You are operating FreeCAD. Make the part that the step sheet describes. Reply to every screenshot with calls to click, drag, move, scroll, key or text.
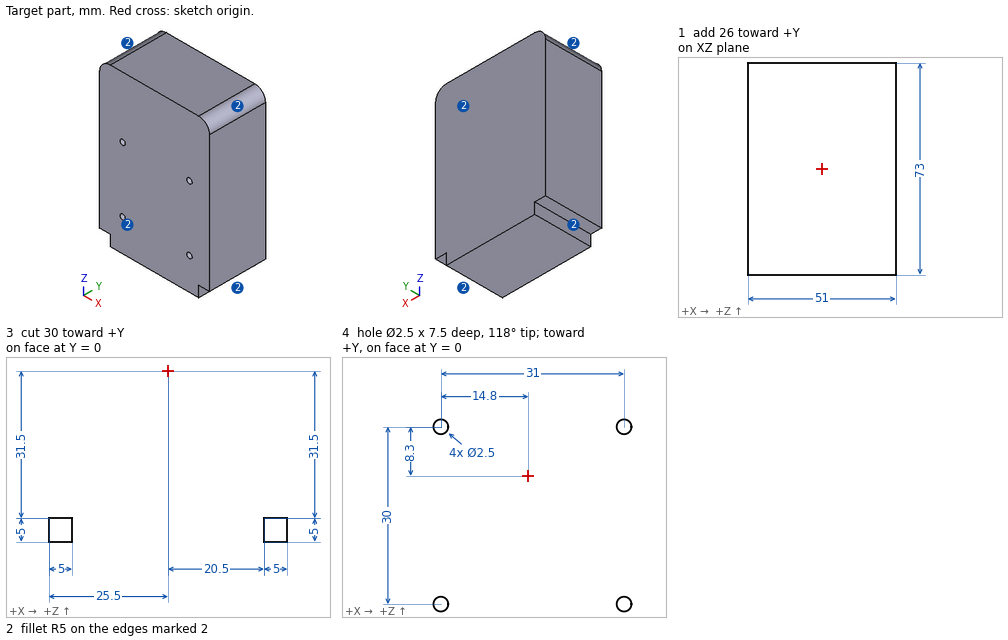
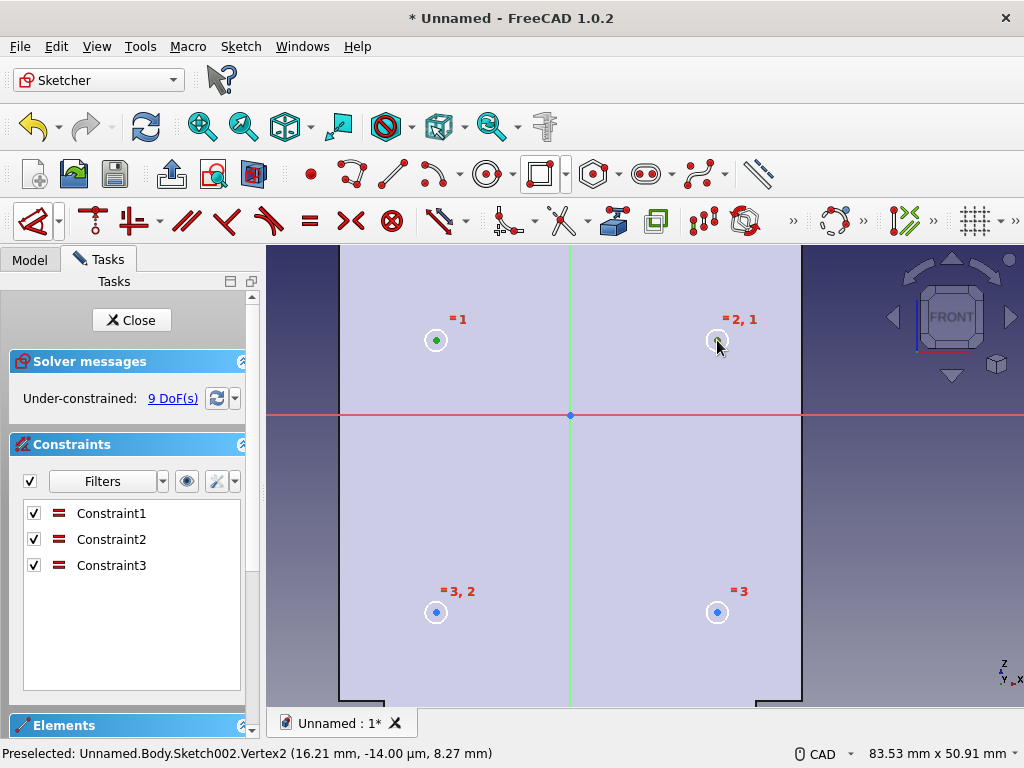
click(160, 222)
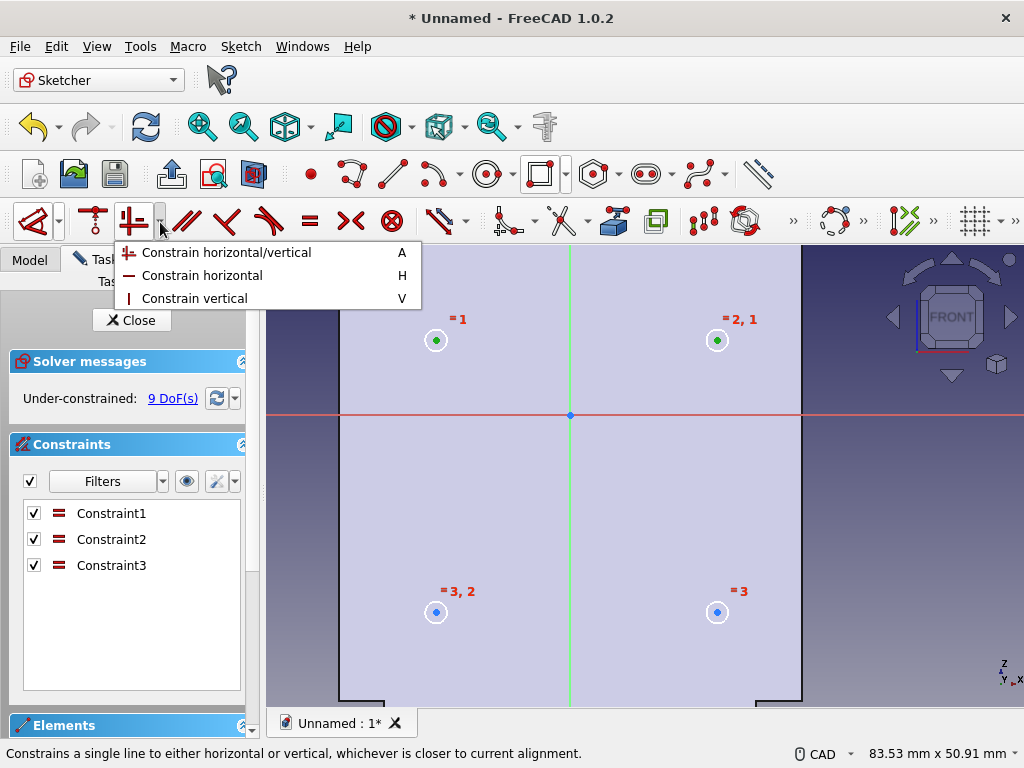
click(268, 276)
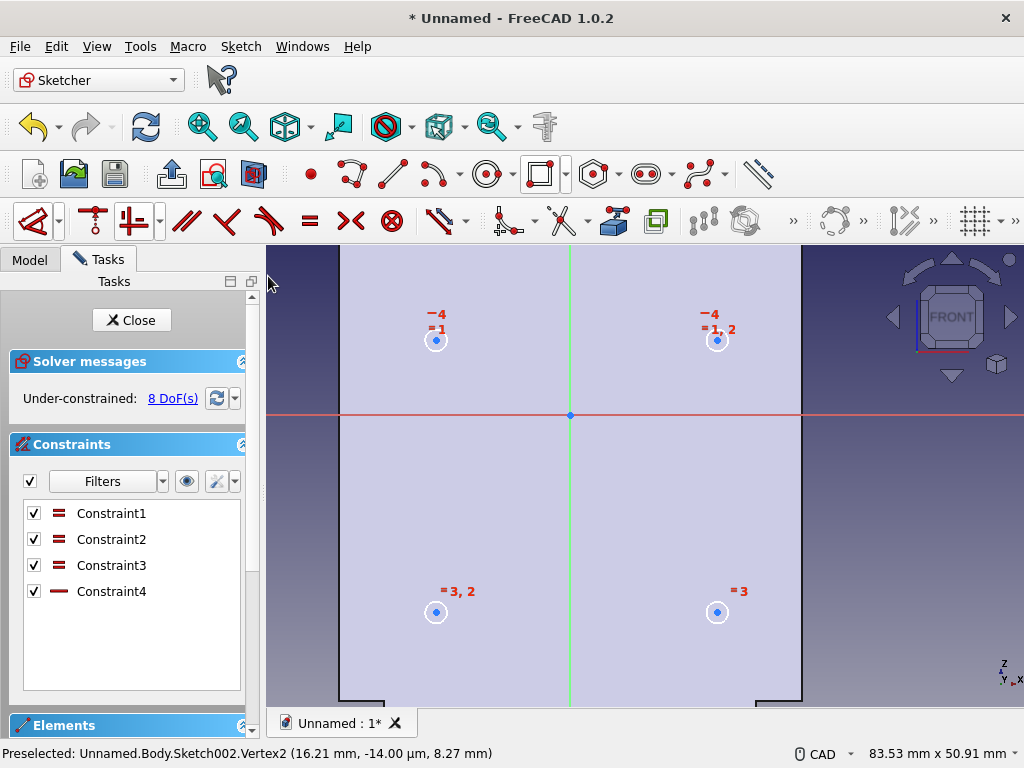
click(436, 340)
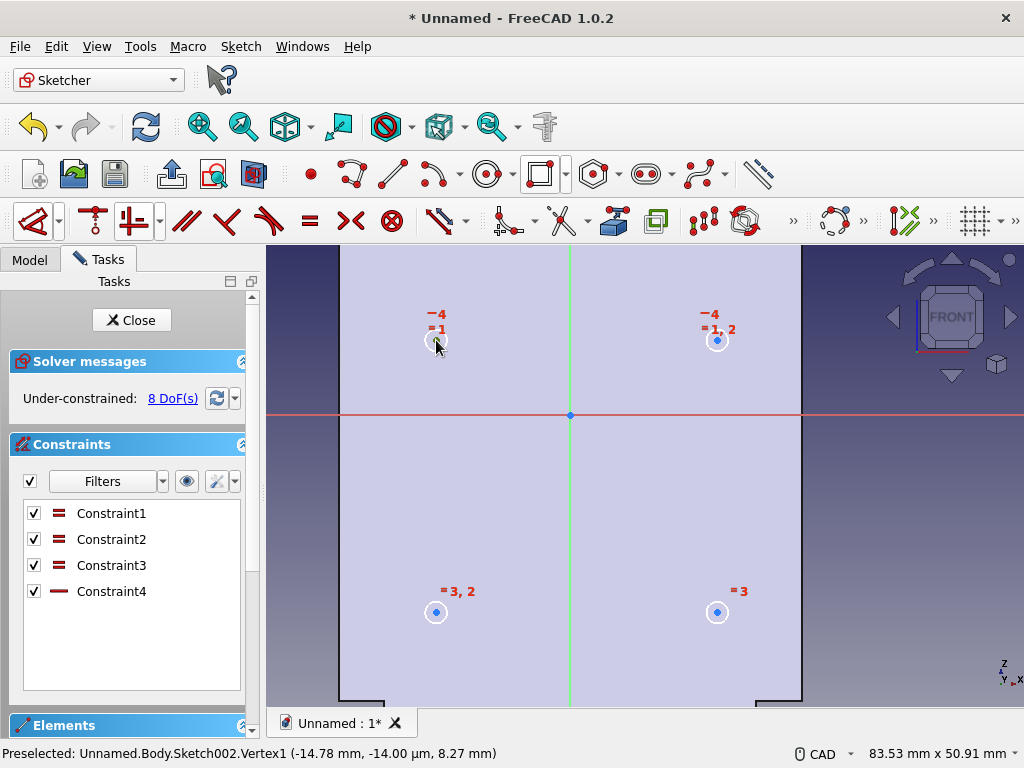
click(436, 613)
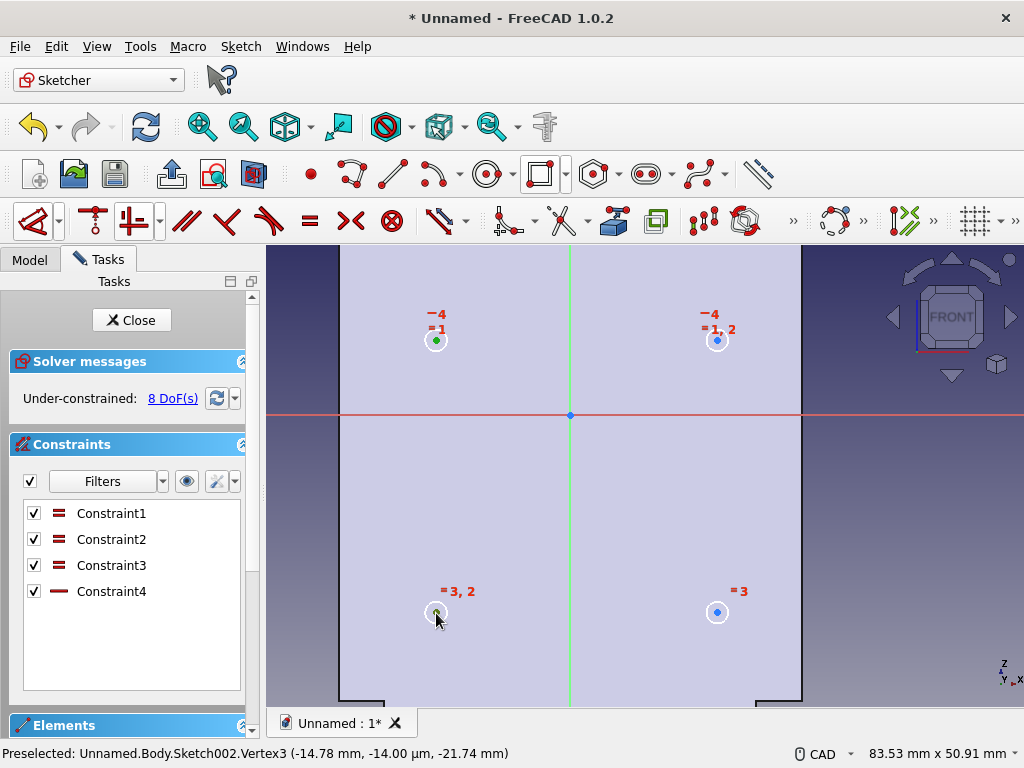
key(v)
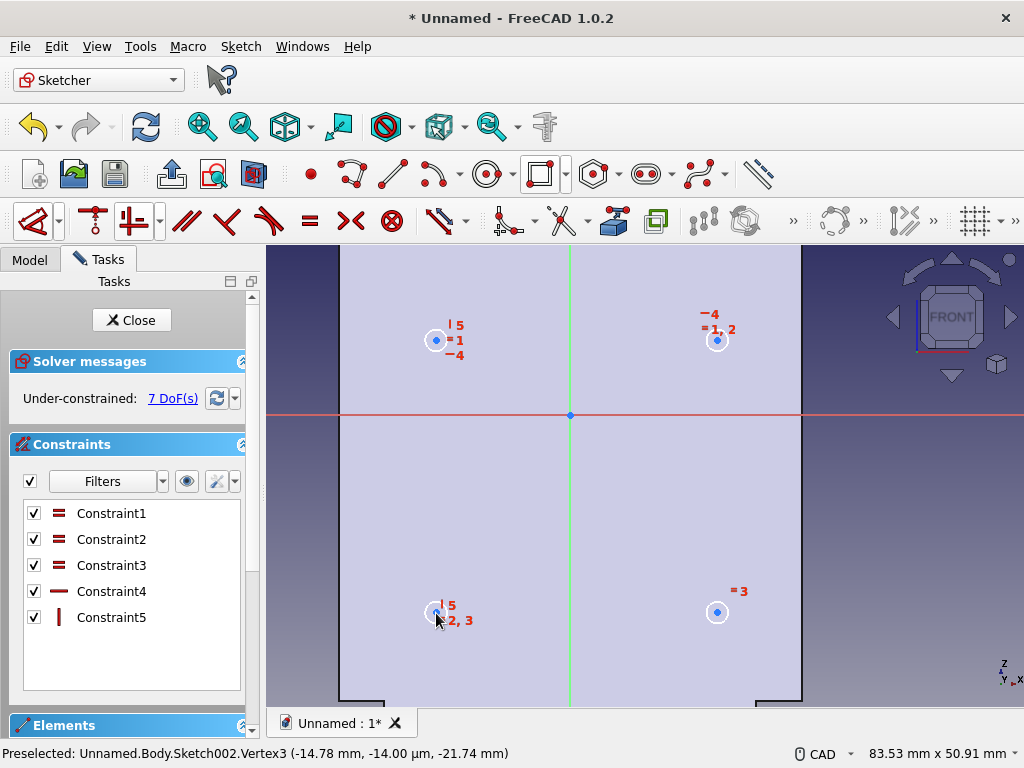
click(717, 340)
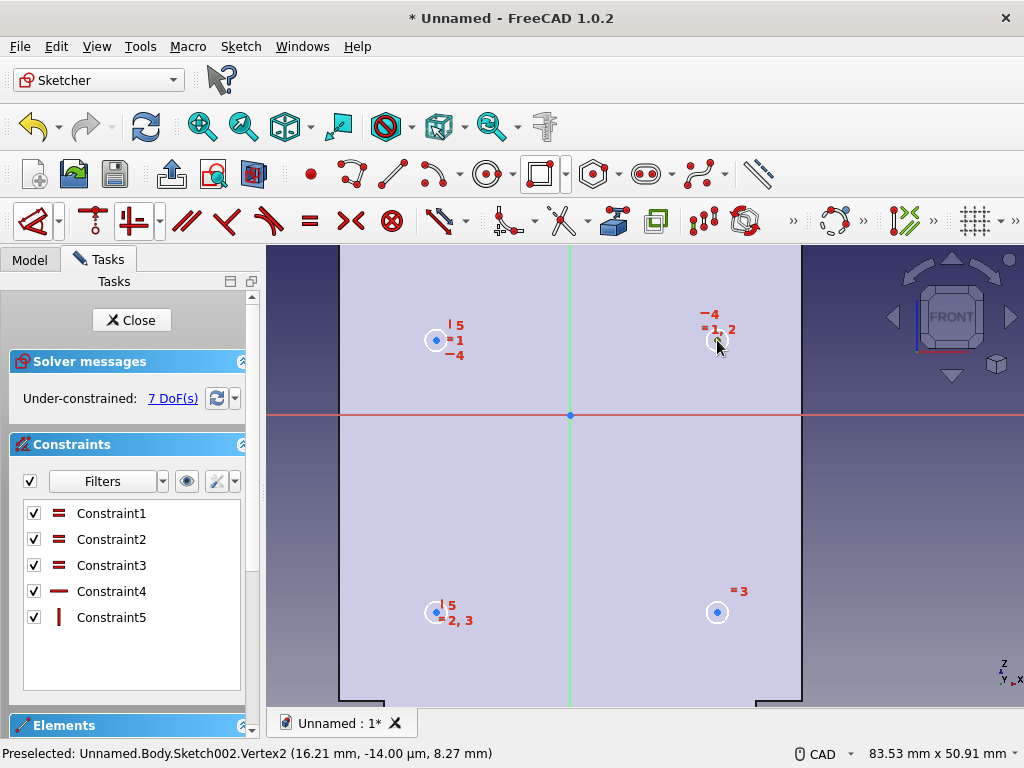
click(717, 613)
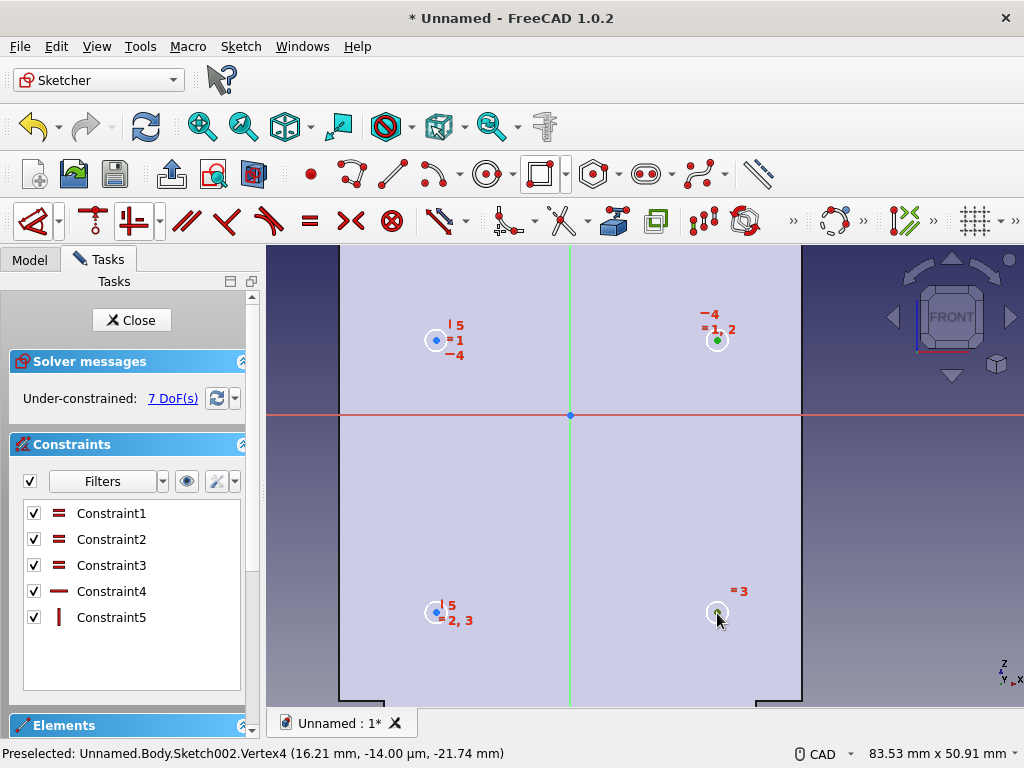
key(v)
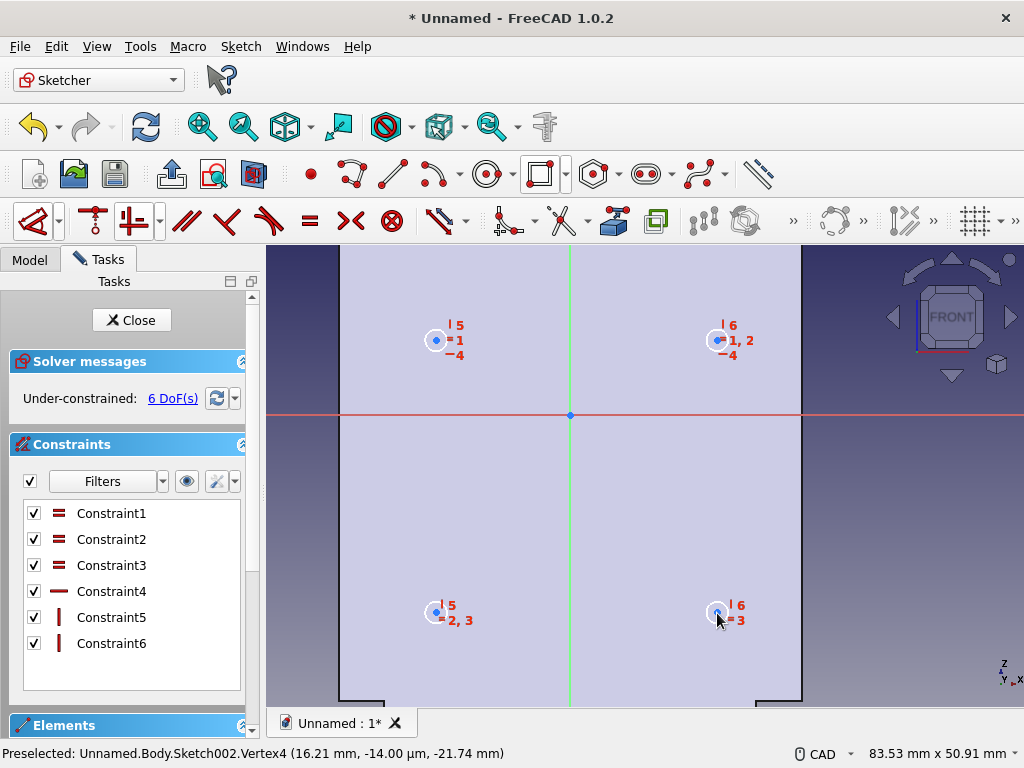
click(436, 613)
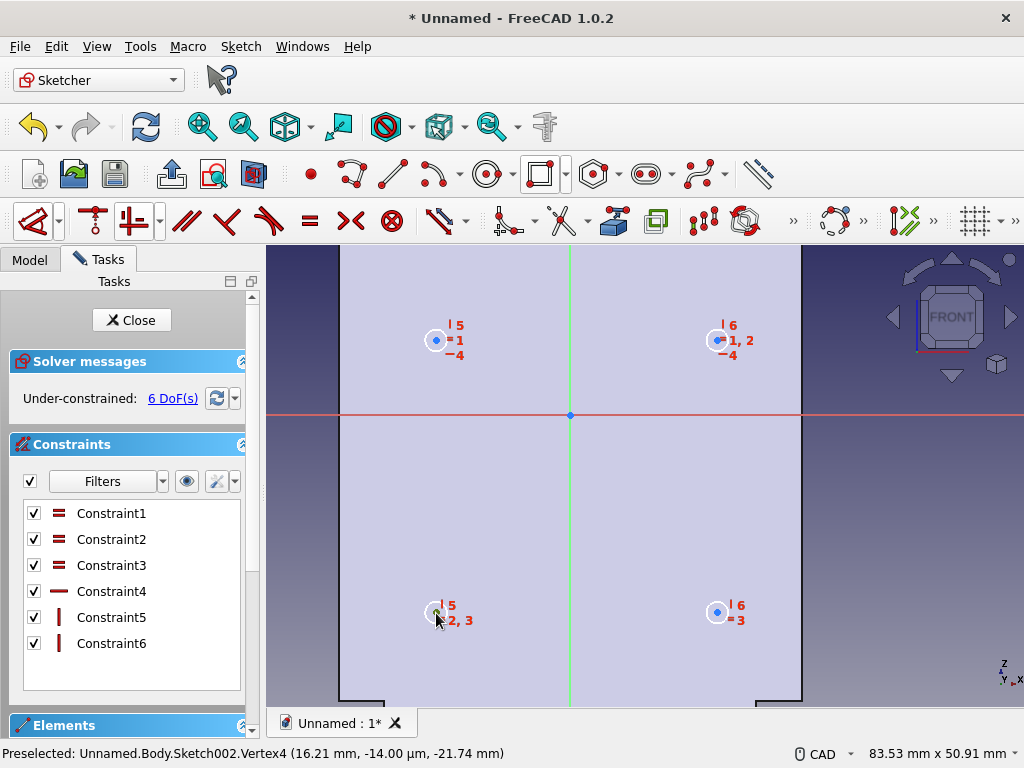
click(717, 613)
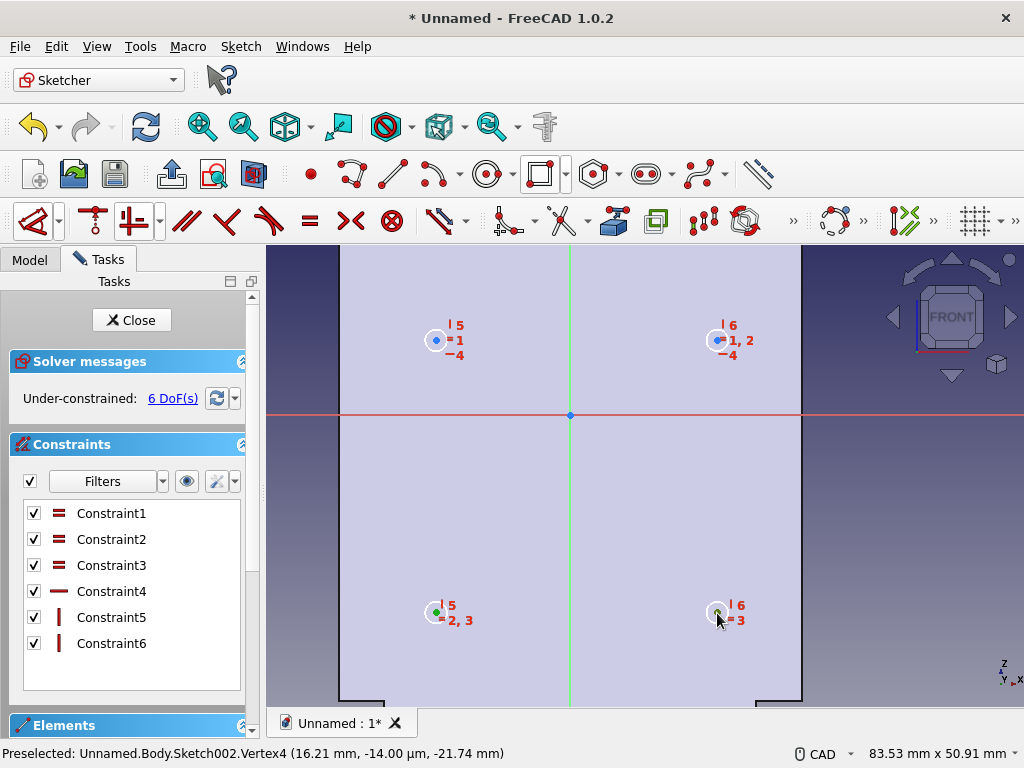
key(h)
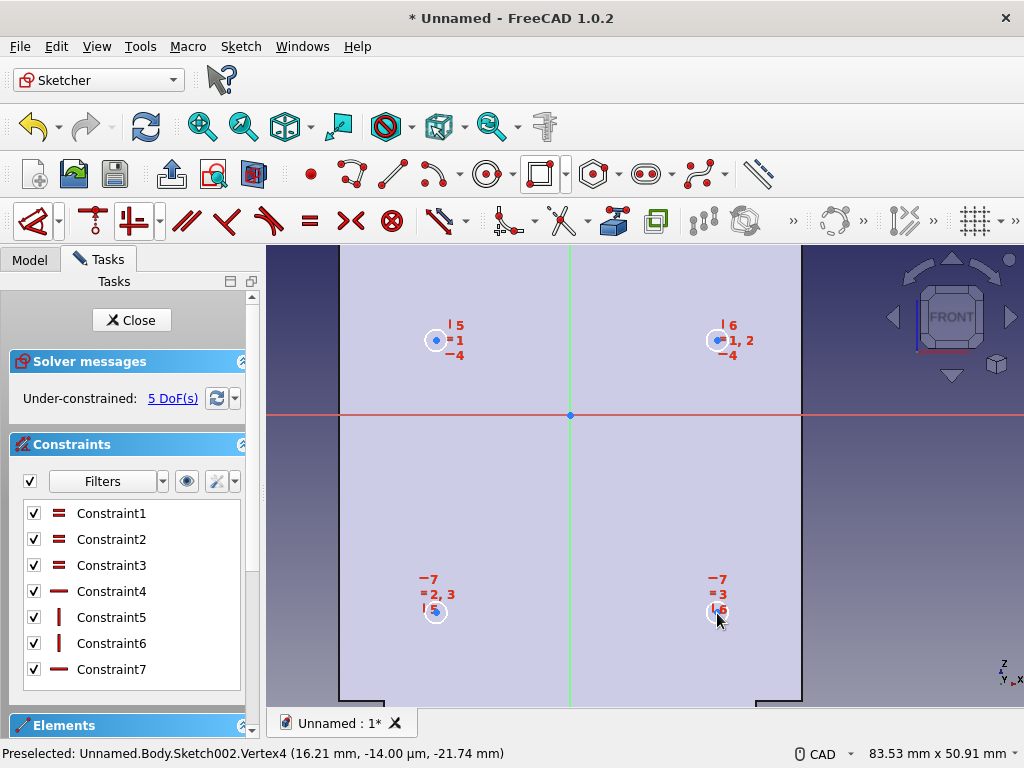
scroll(444, 333, up, 3)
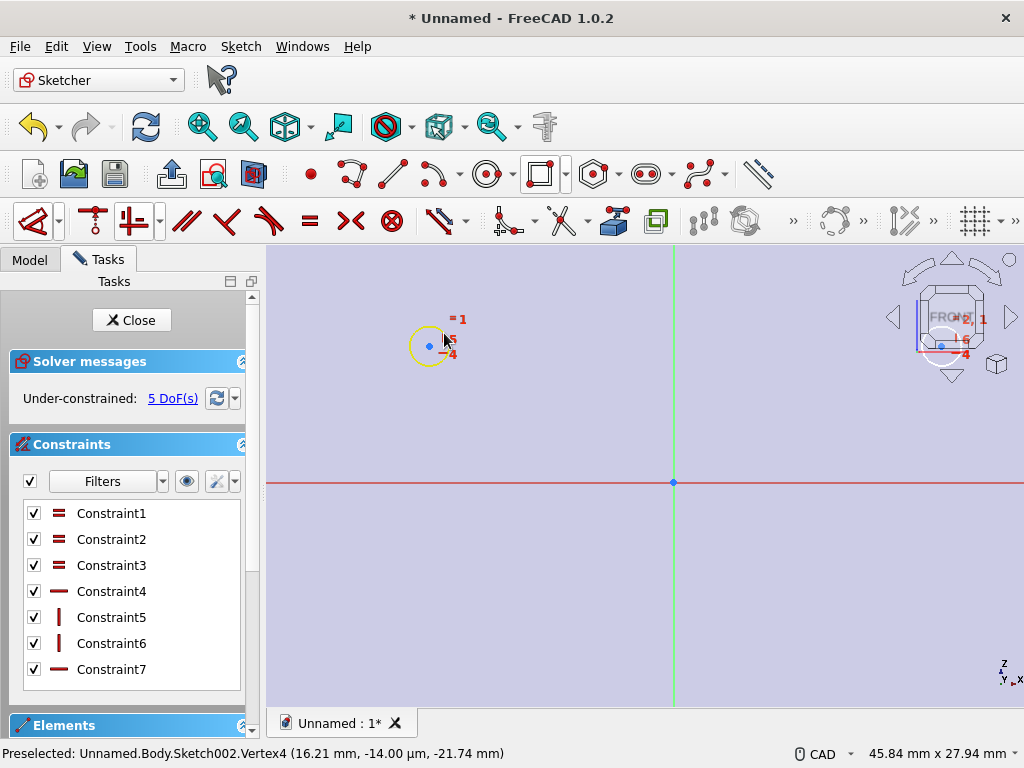
click(415, 332)